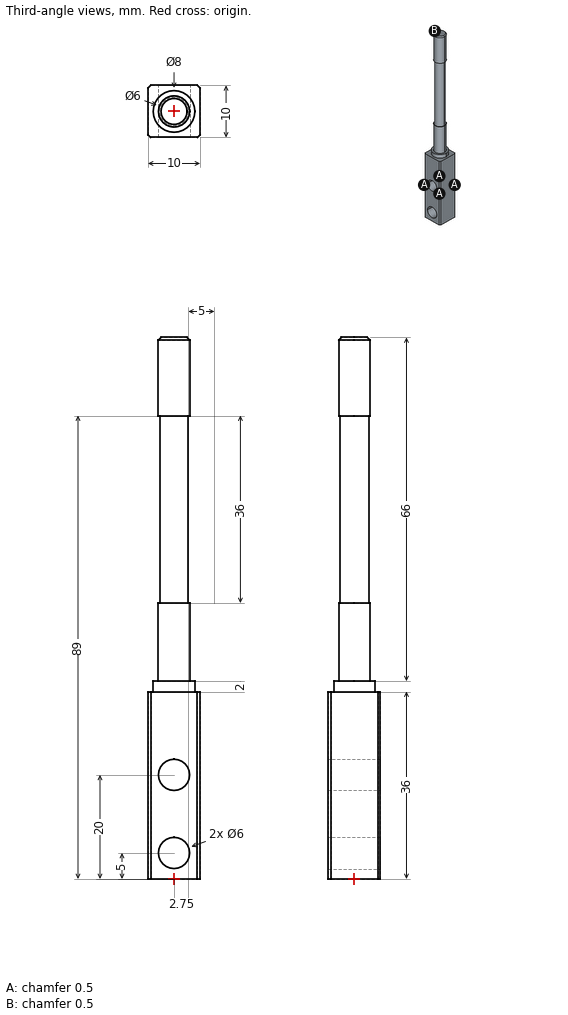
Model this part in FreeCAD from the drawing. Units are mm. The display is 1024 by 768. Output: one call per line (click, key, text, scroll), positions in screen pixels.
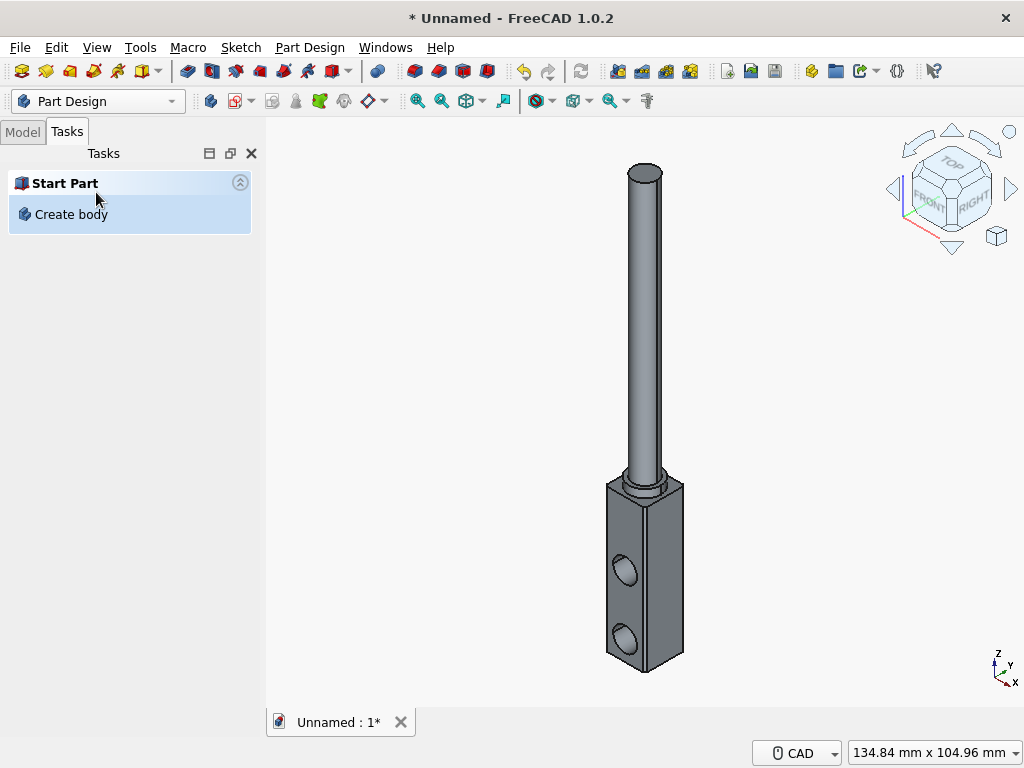
click(628, 171)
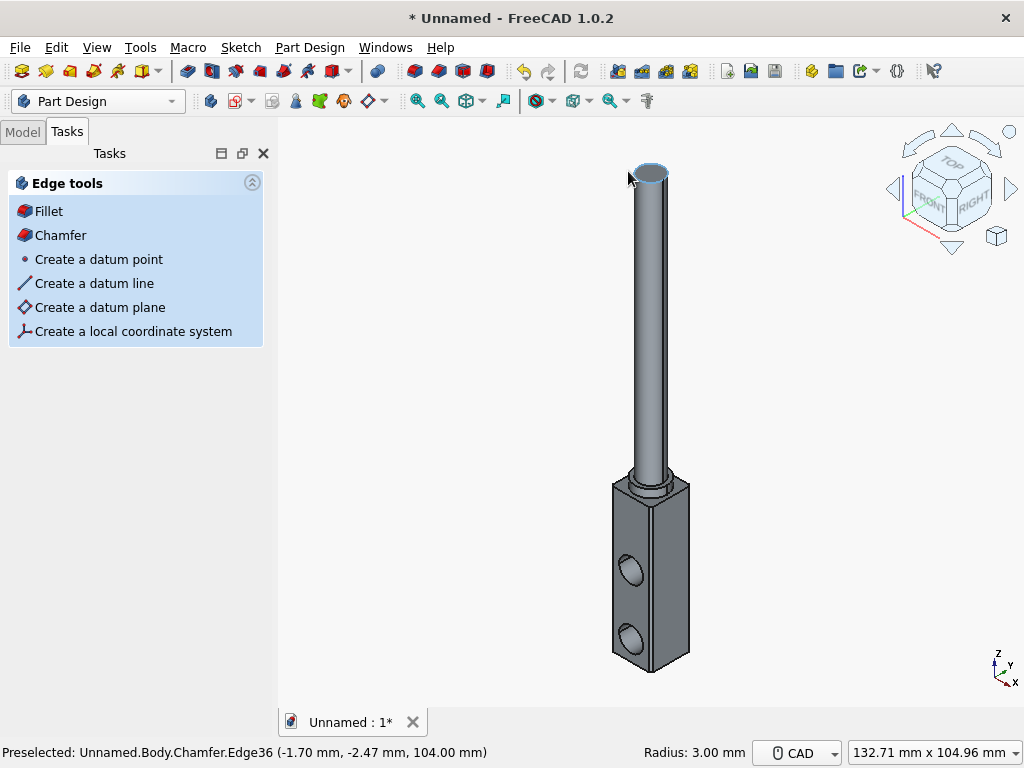
click(440, 72)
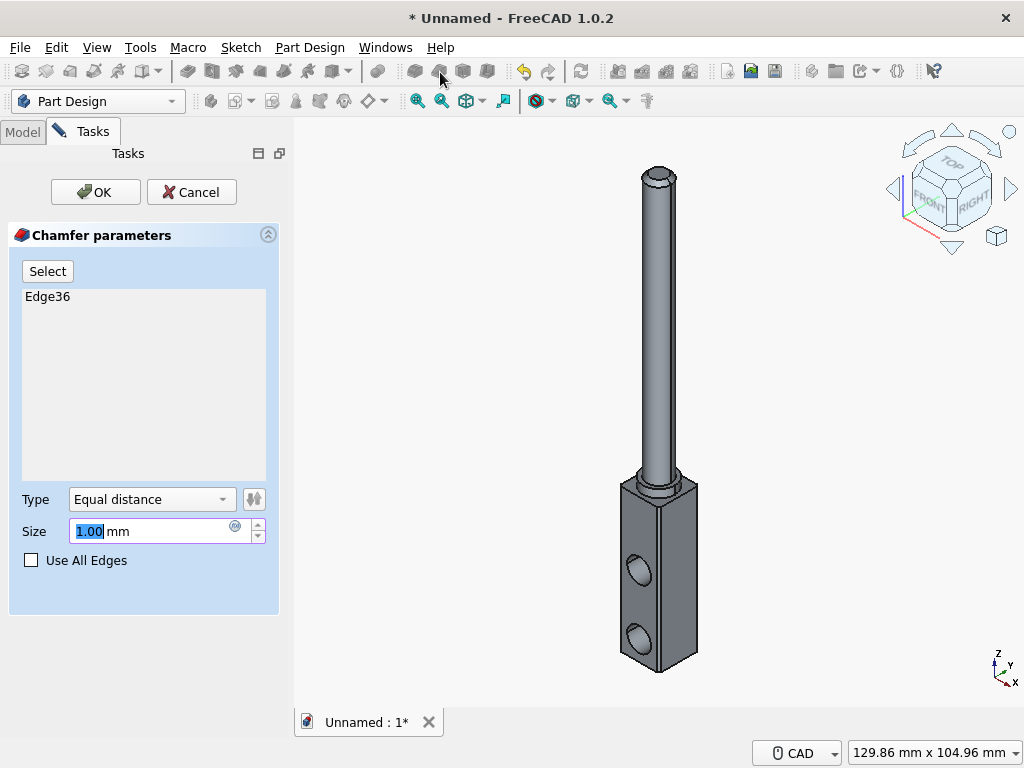
text(0.5)
key(Tab)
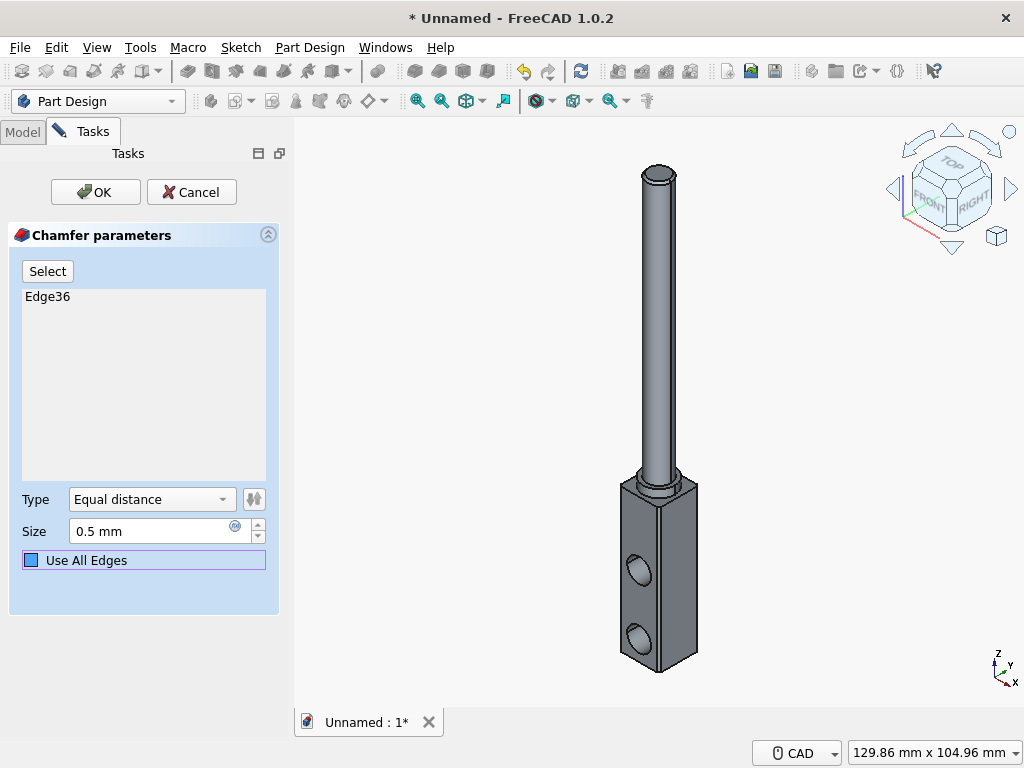
click(96, 192)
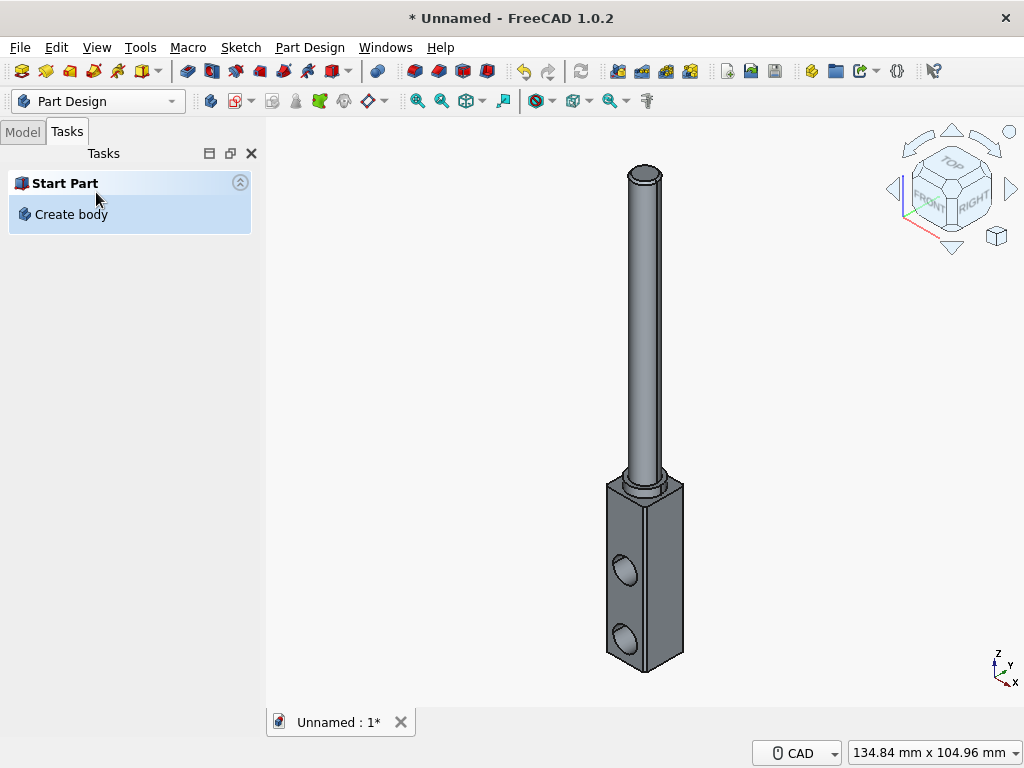
click(236, 102)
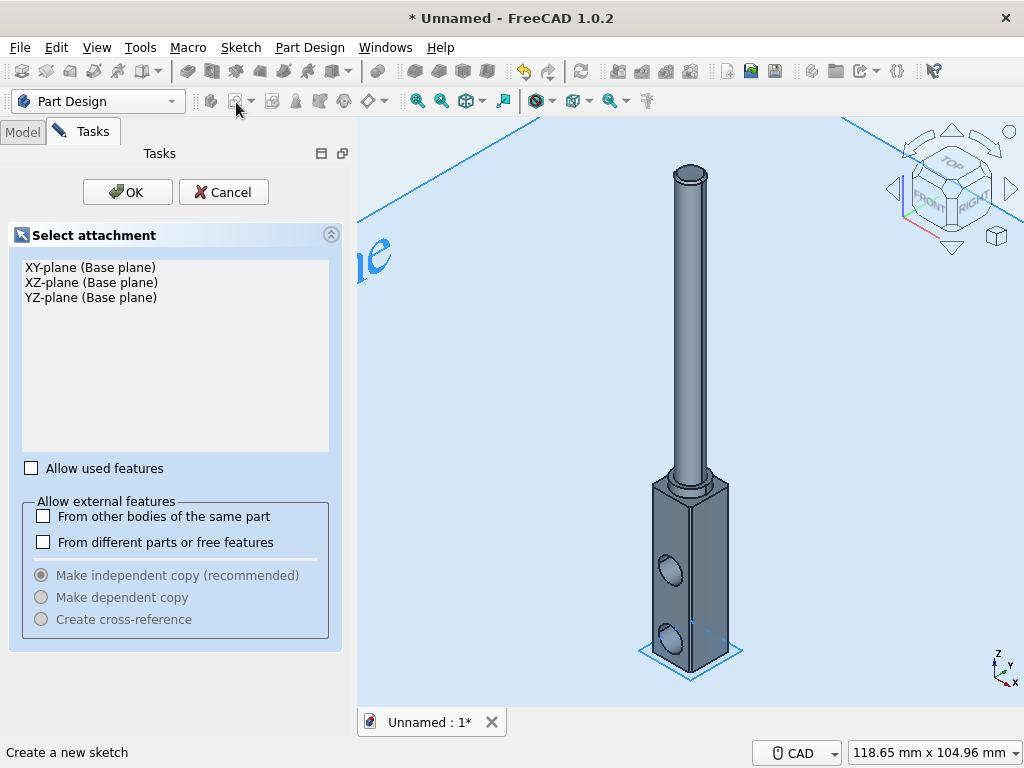
click(82, 282)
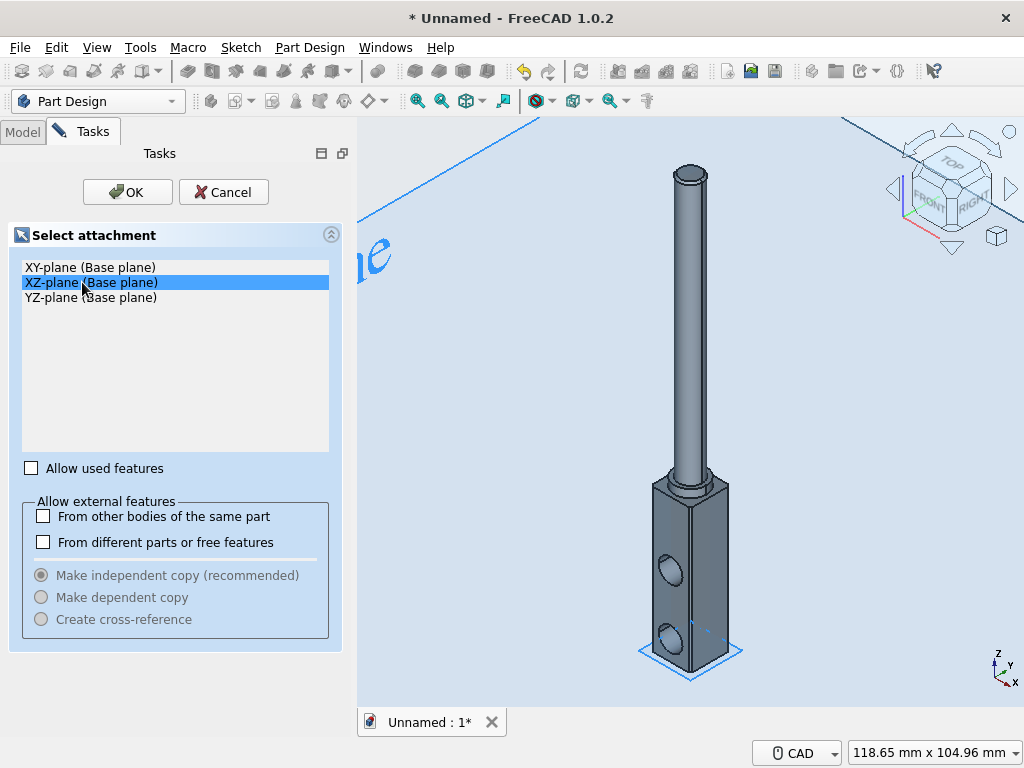
click(128, 192)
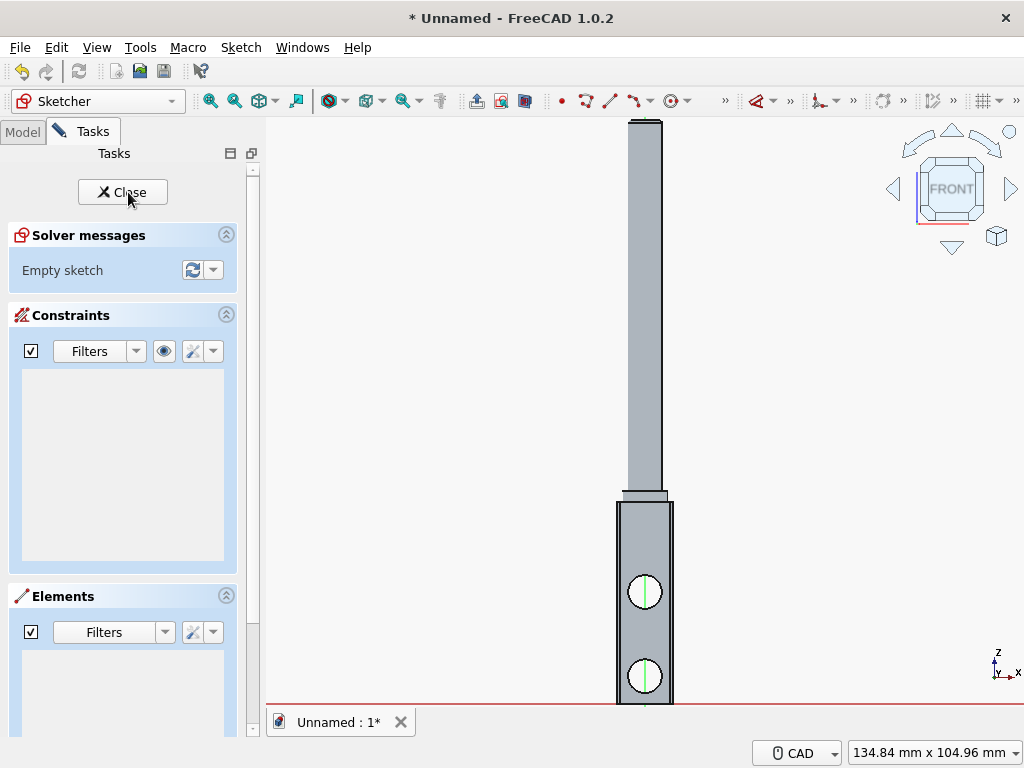
click(526, 102)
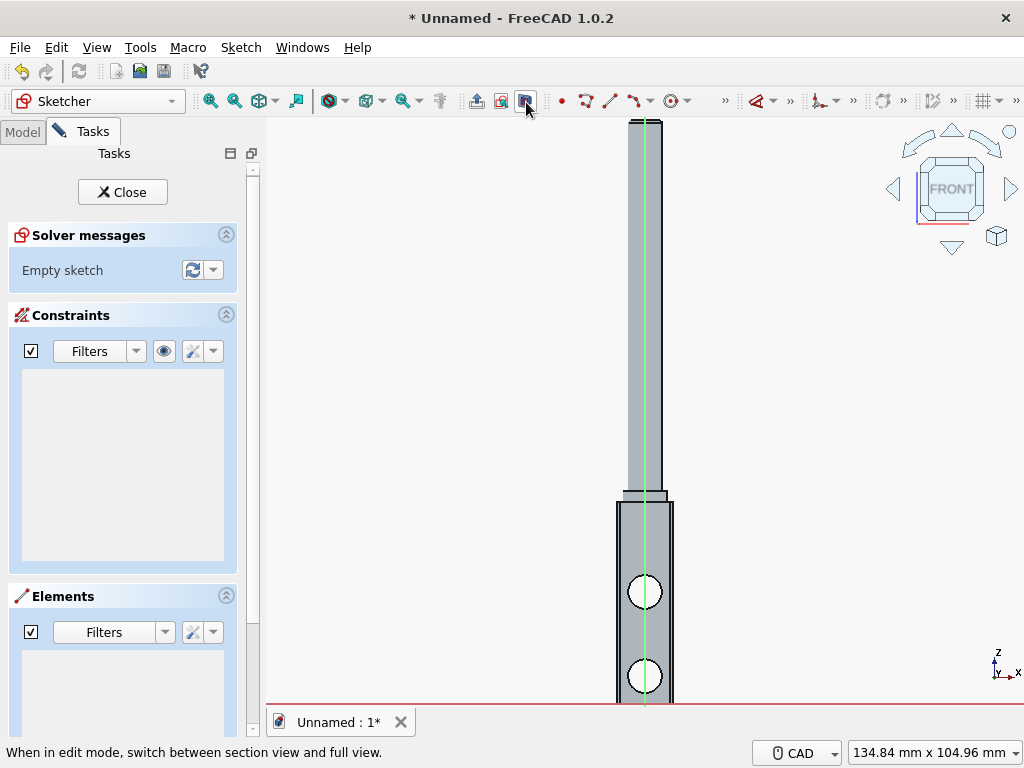
scroll(294, 222, down, 1)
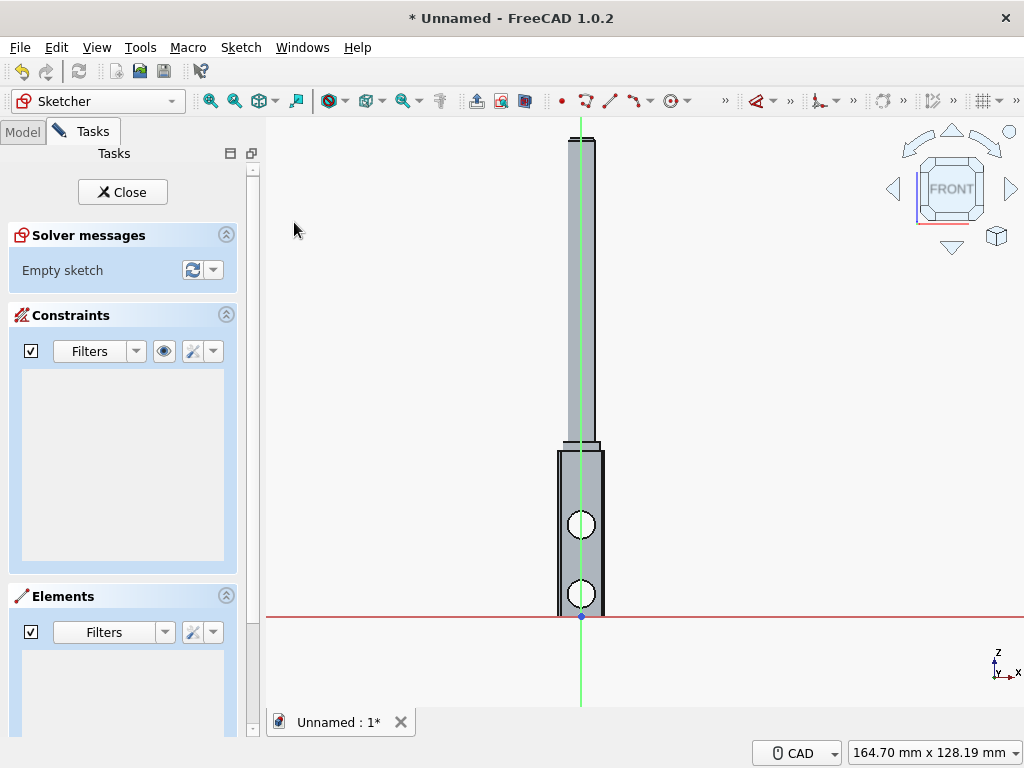
key(g)
key(r)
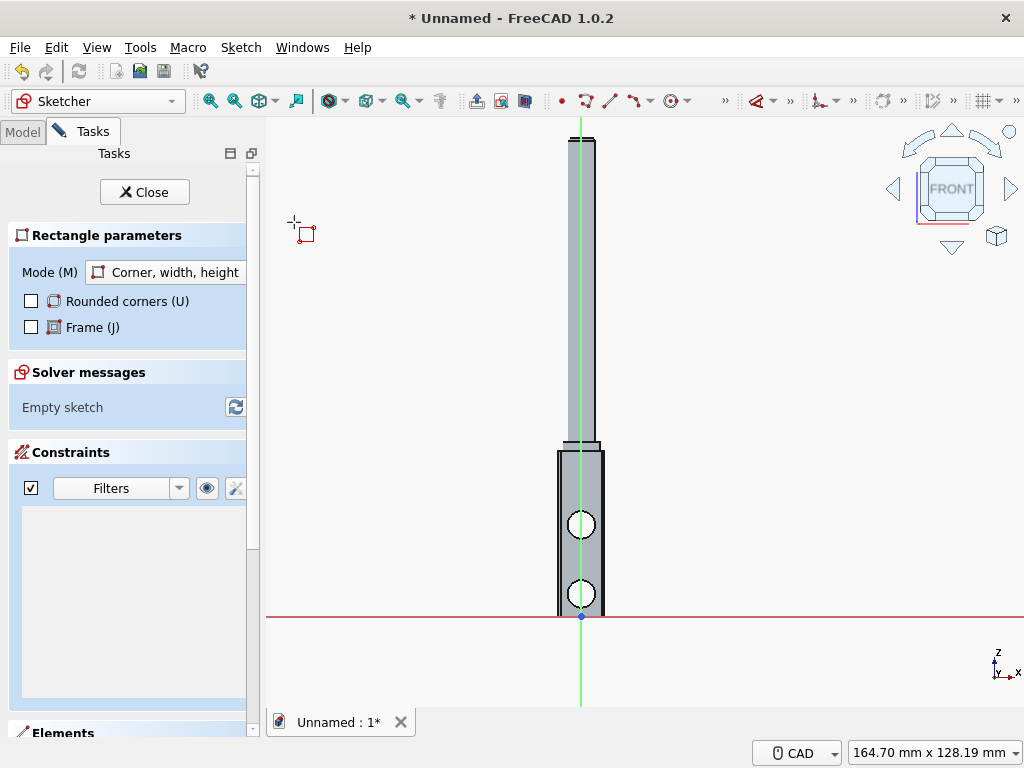
scroll(594, 207, up, 2)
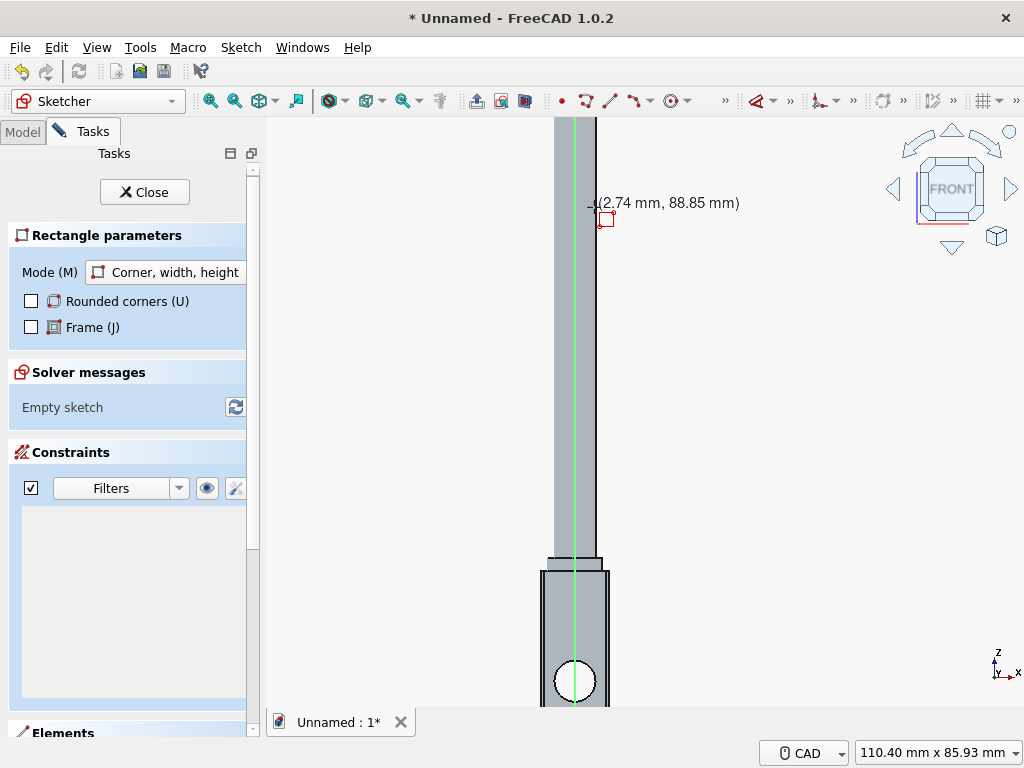
click(594, 207)
click(628, 455)
key(Escape)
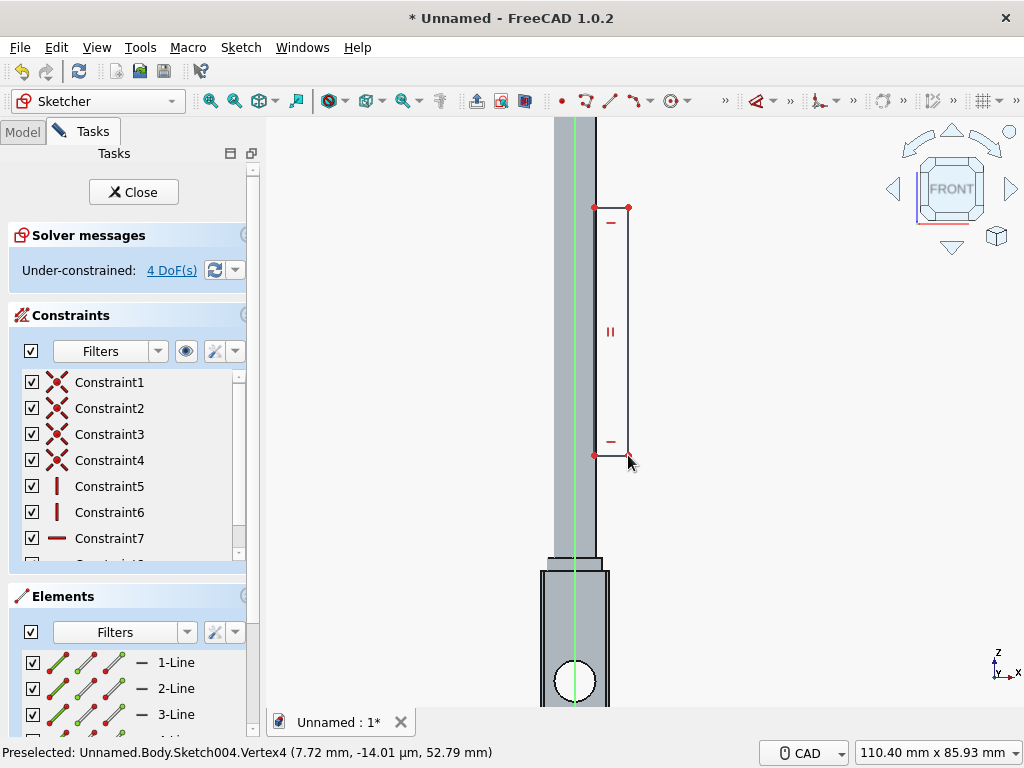
key(d)